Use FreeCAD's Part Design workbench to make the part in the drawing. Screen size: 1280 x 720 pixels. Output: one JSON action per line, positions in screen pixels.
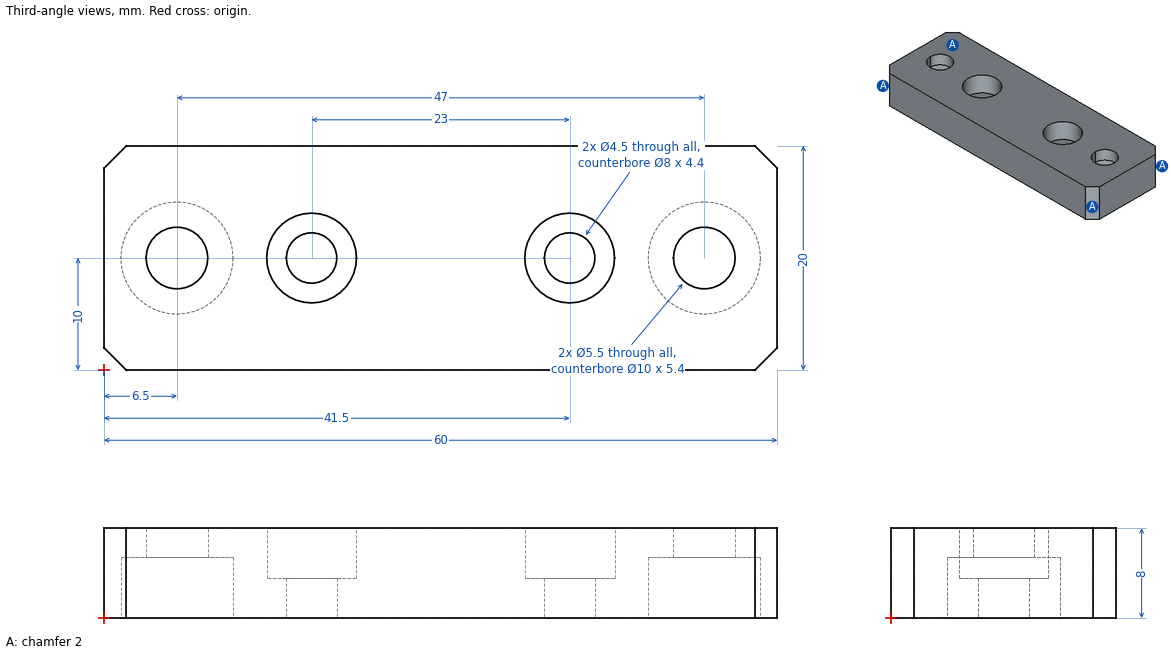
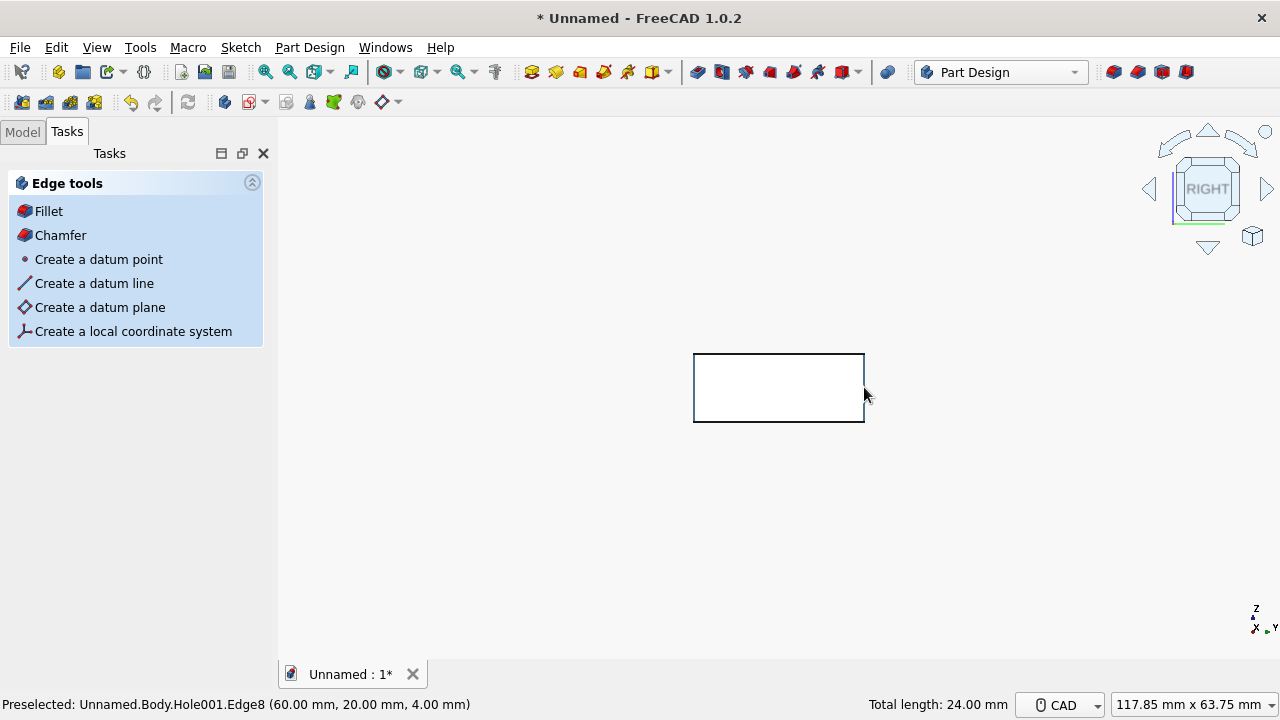
{"action": "key", "text": "5"}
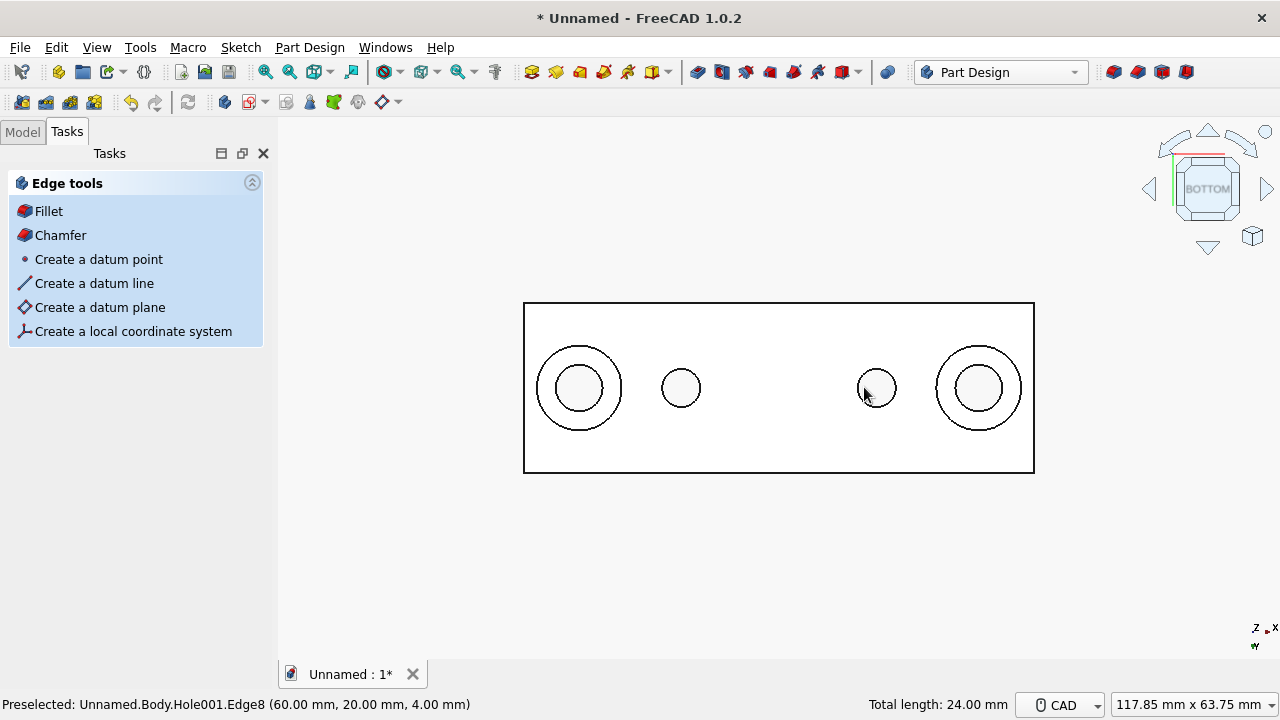
{"action": "key", "text": "4"}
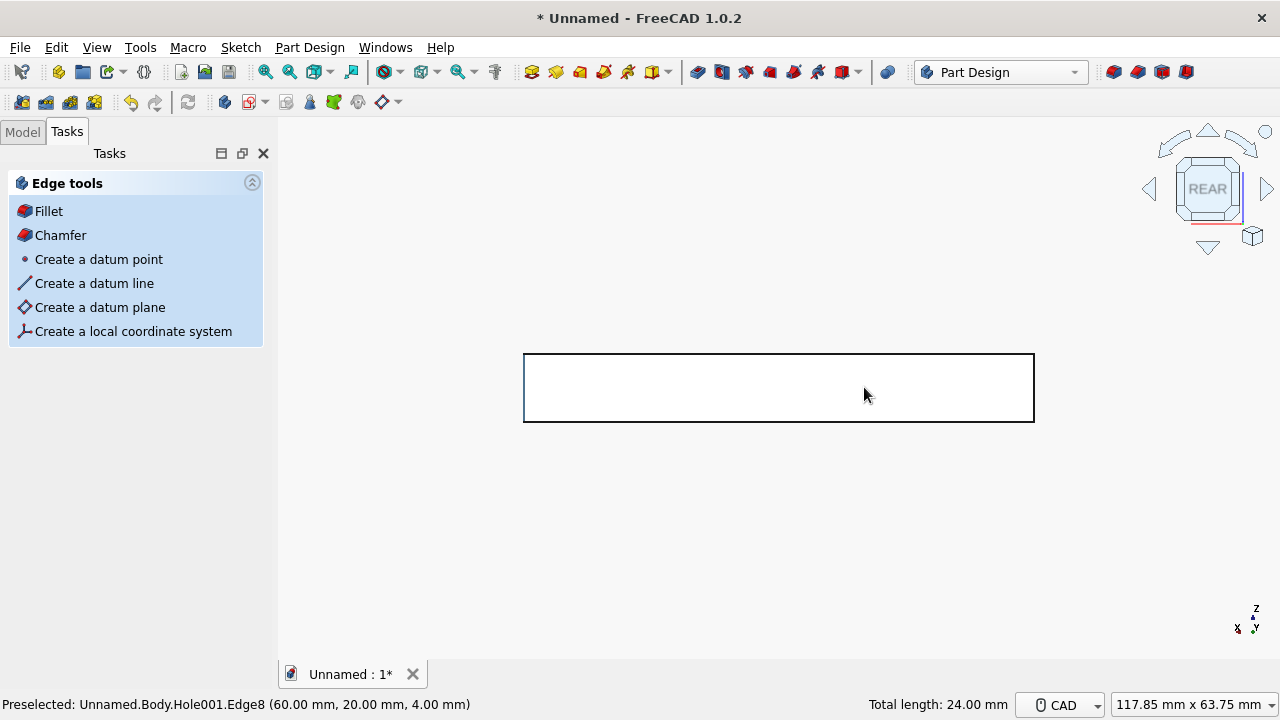
{"action": "left_click", "coordinate": [1034, 387], "text": "ctrl"}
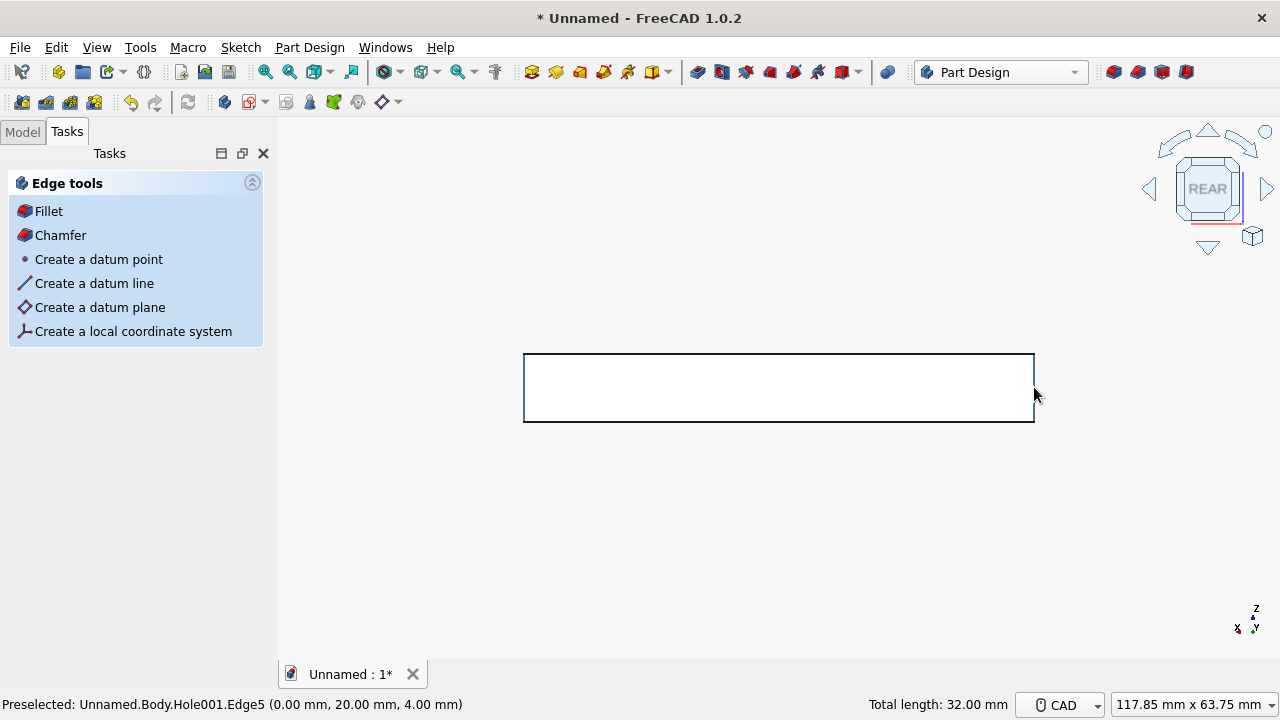
{"action": "left_click", "coordinate": [1138, 72]}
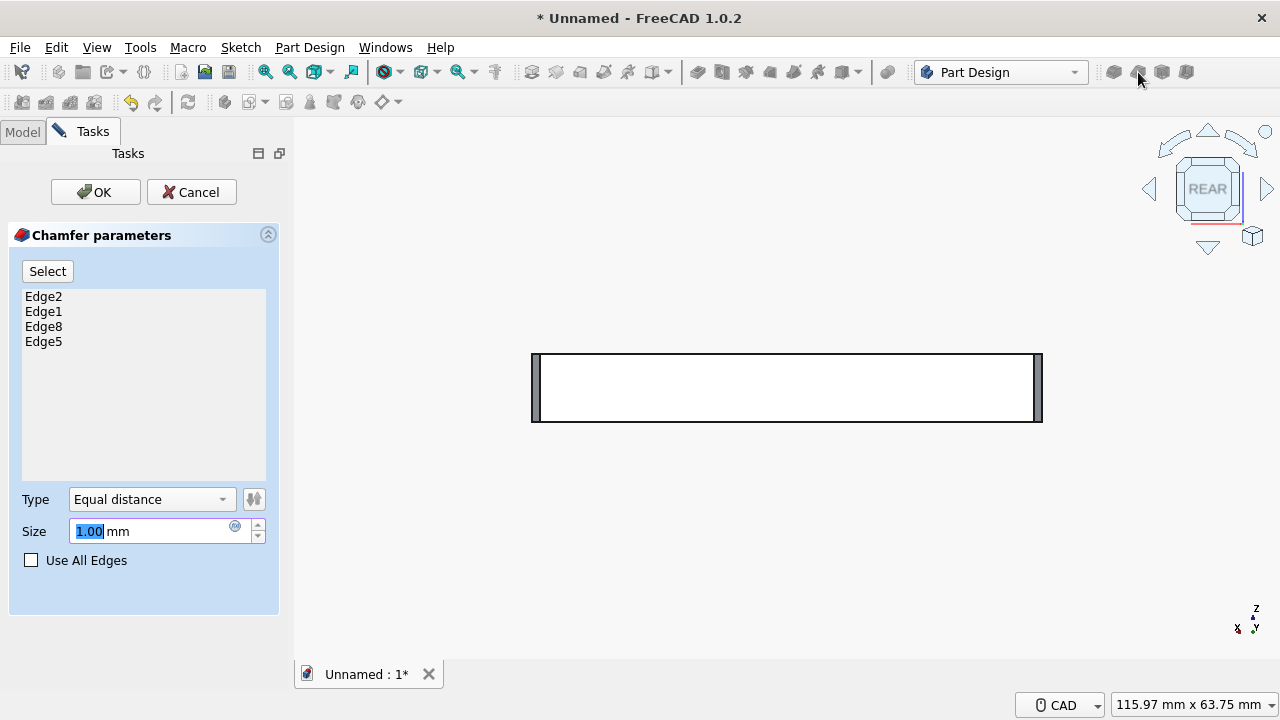
{"action": "type", "text": "2"}
{"action": "key", "text": "Tab"}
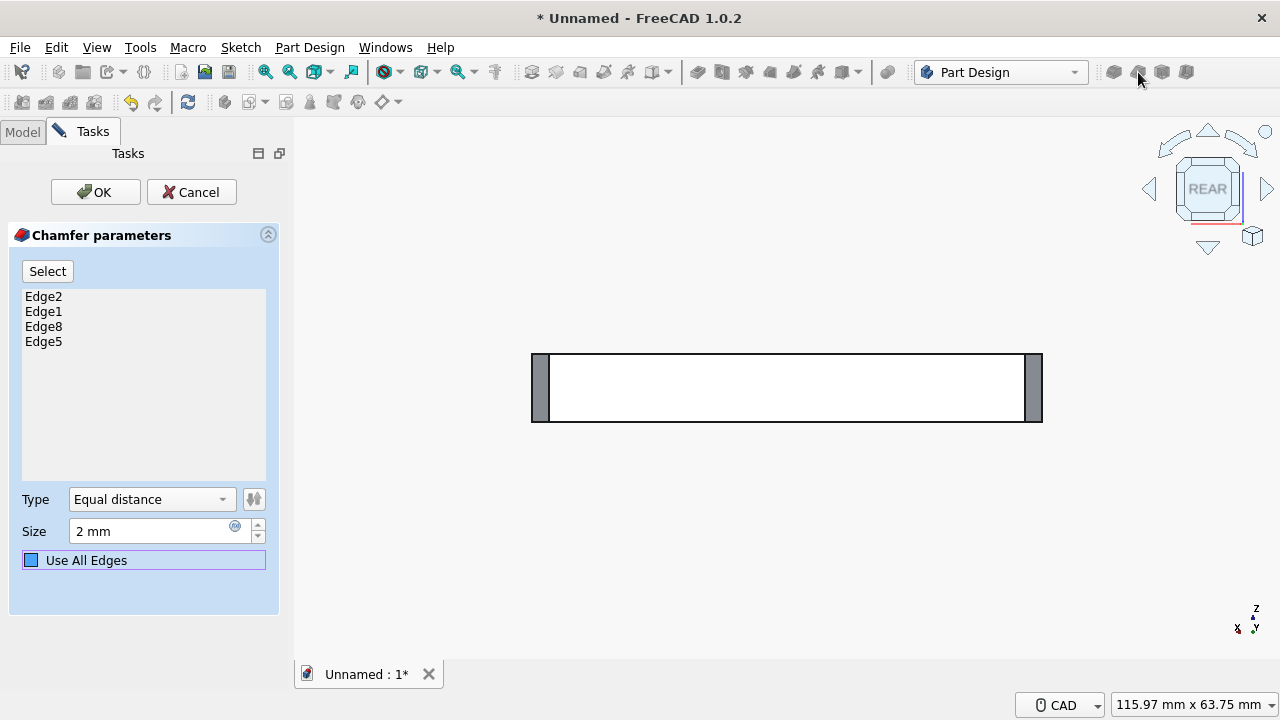
{"action": "left_click", "coordinate": [96, 192]}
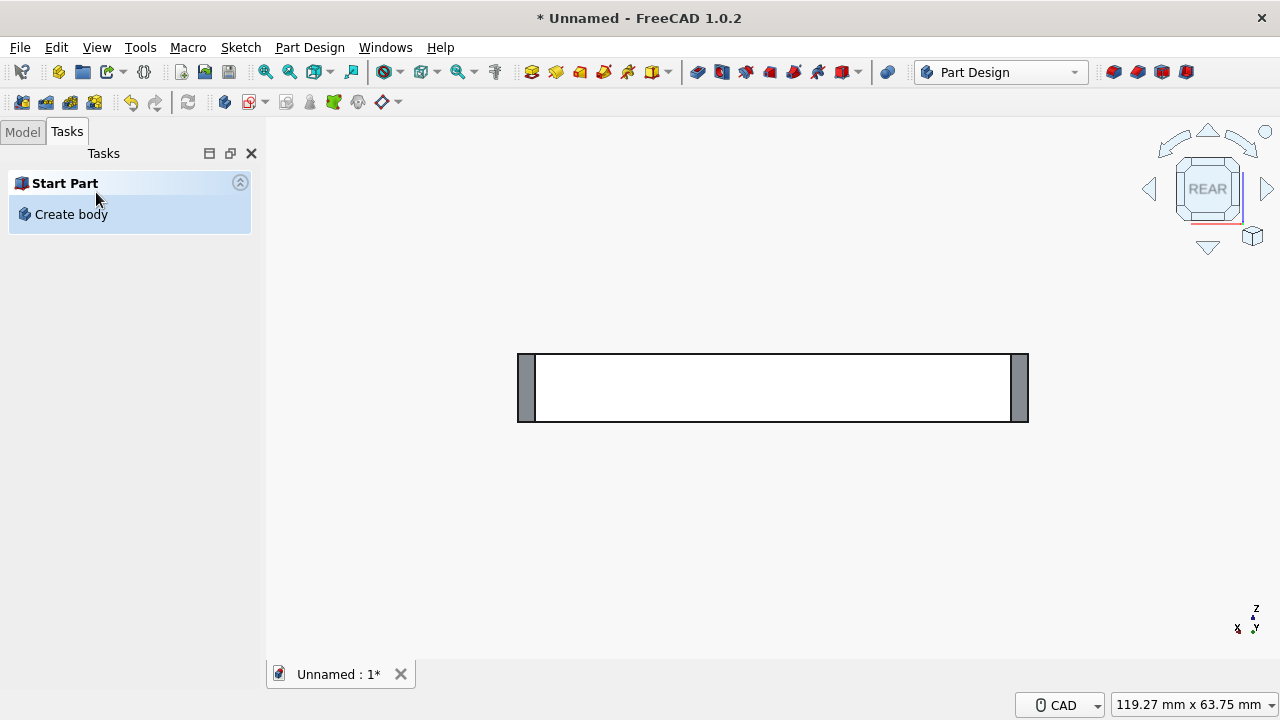
{"action": "key", "text": "0"}